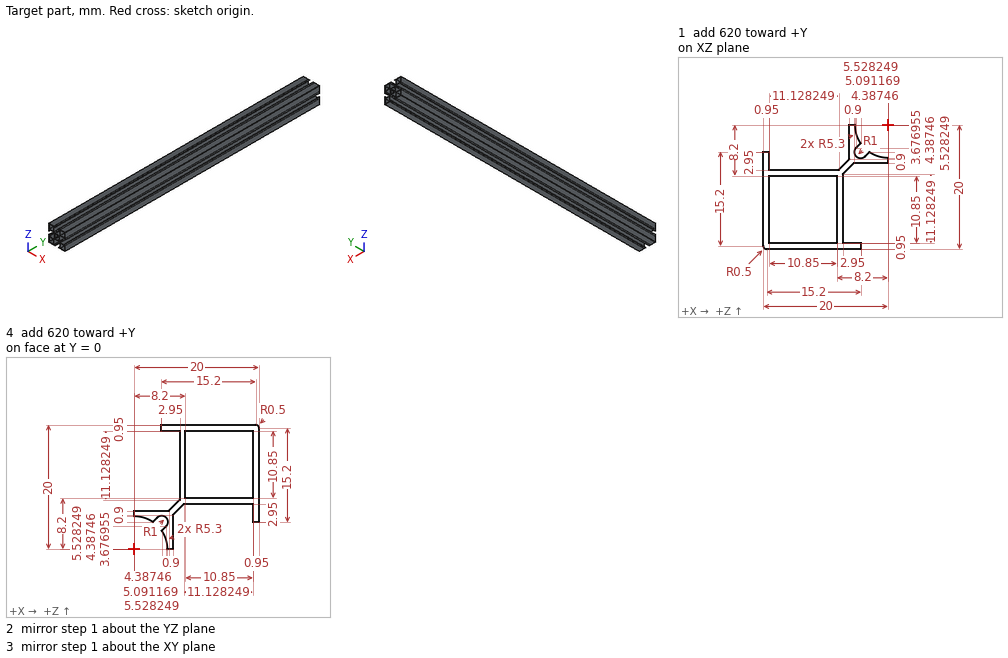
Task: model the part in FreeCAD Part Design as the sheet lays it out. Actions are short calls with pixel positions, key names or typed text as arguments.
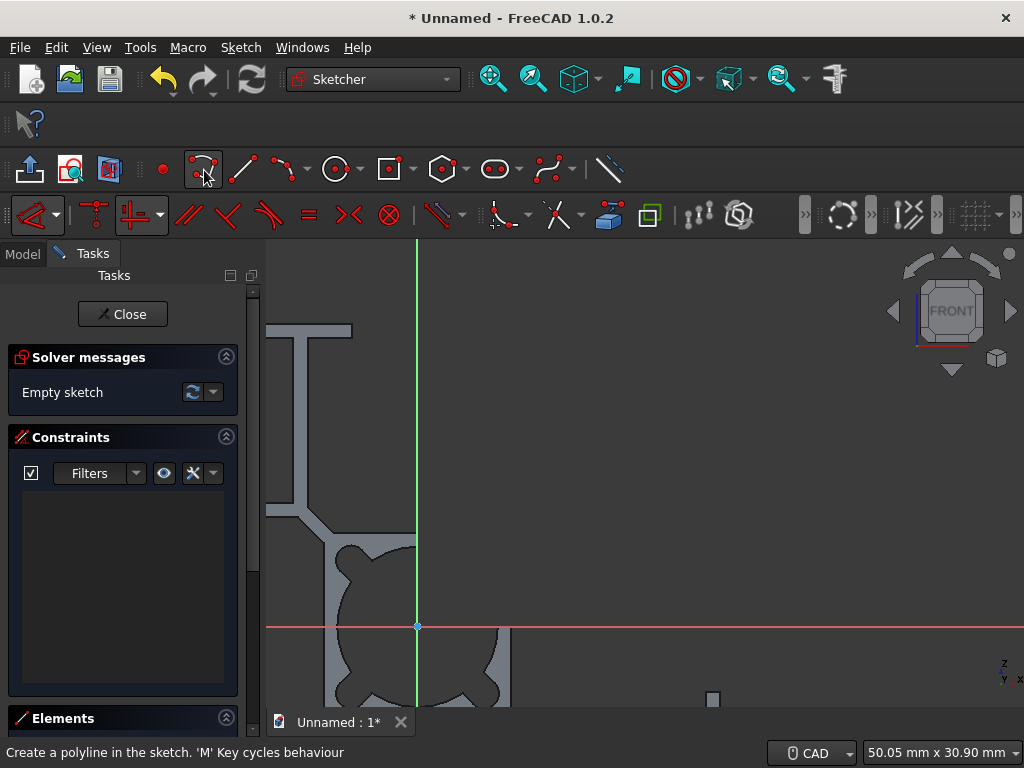
click(720, 332)
click(720, 562)
click(706, 562)
click(706, 517)
click(537, 517)
click(511, 543)
click(511, 627)
click(498, 618)
right_click(498, 618)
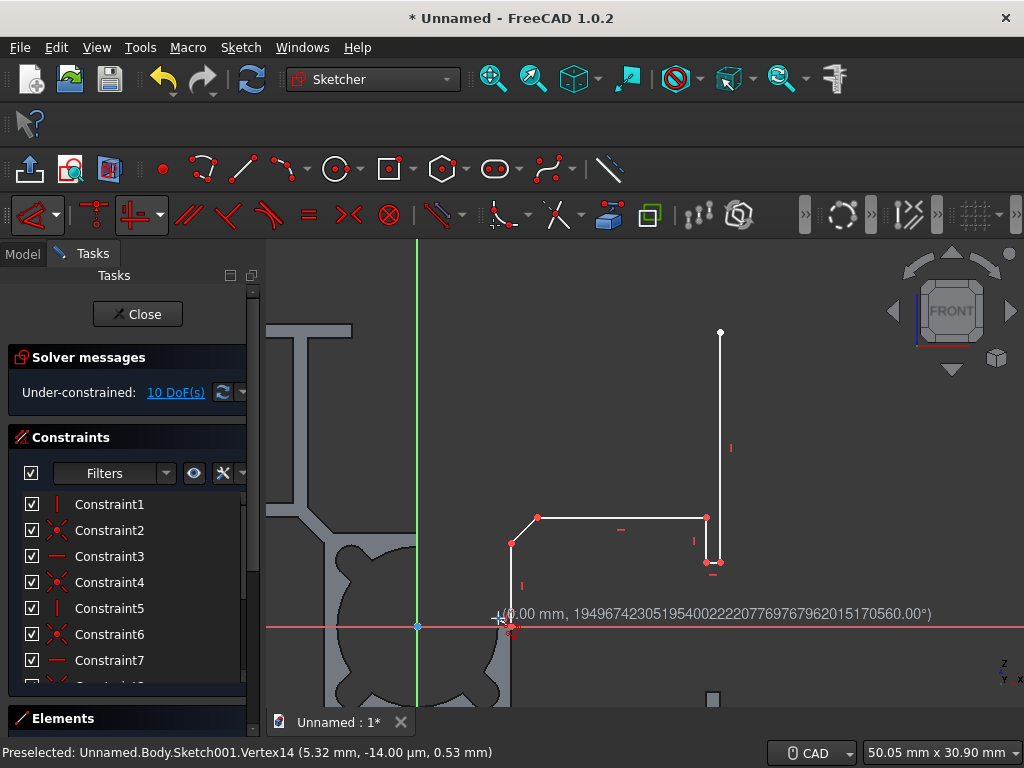
click(244, 170)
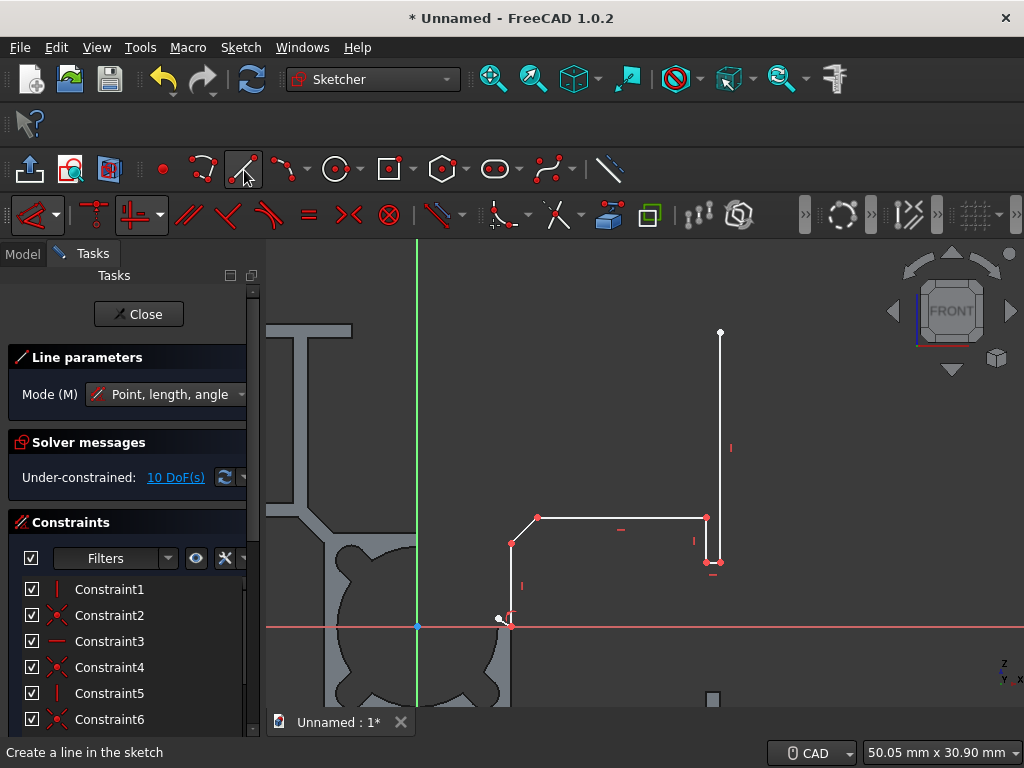
click(484, 582)
click(495, 571)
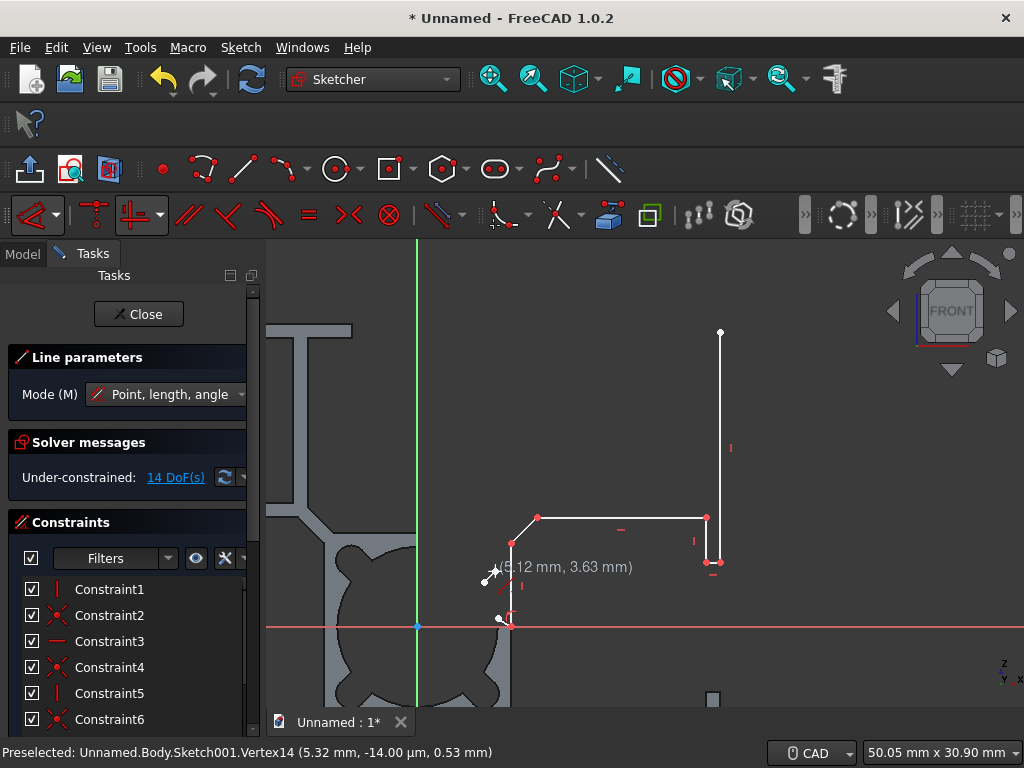
click(473, 550)
click(463, 561)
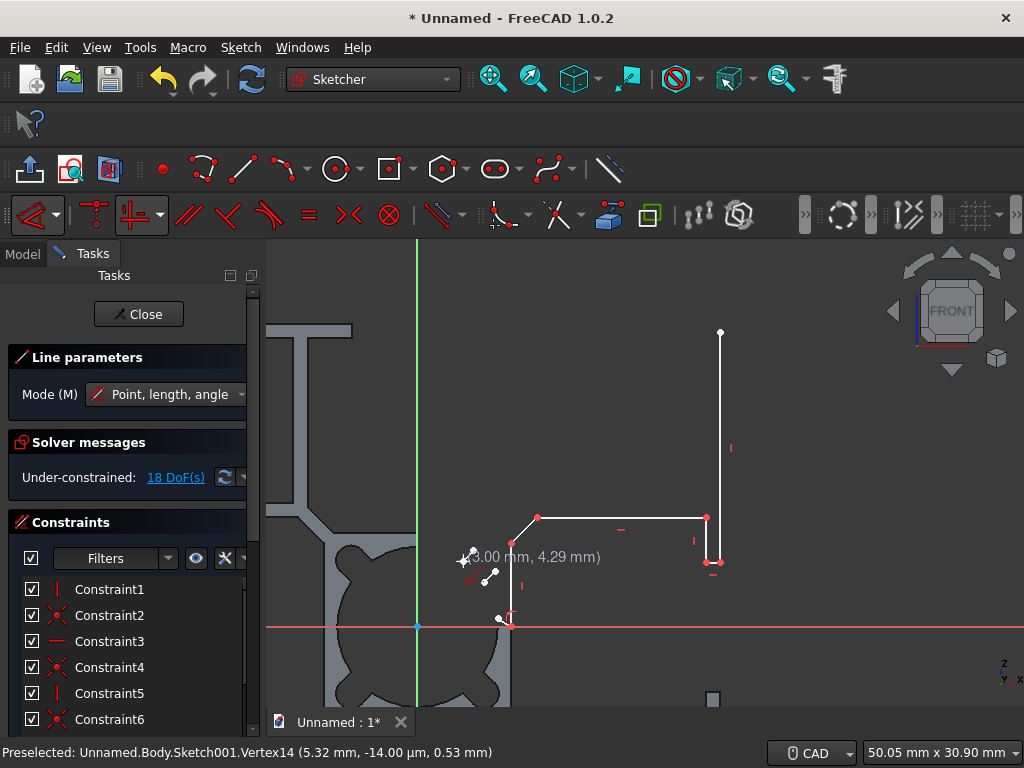
click(204, 170)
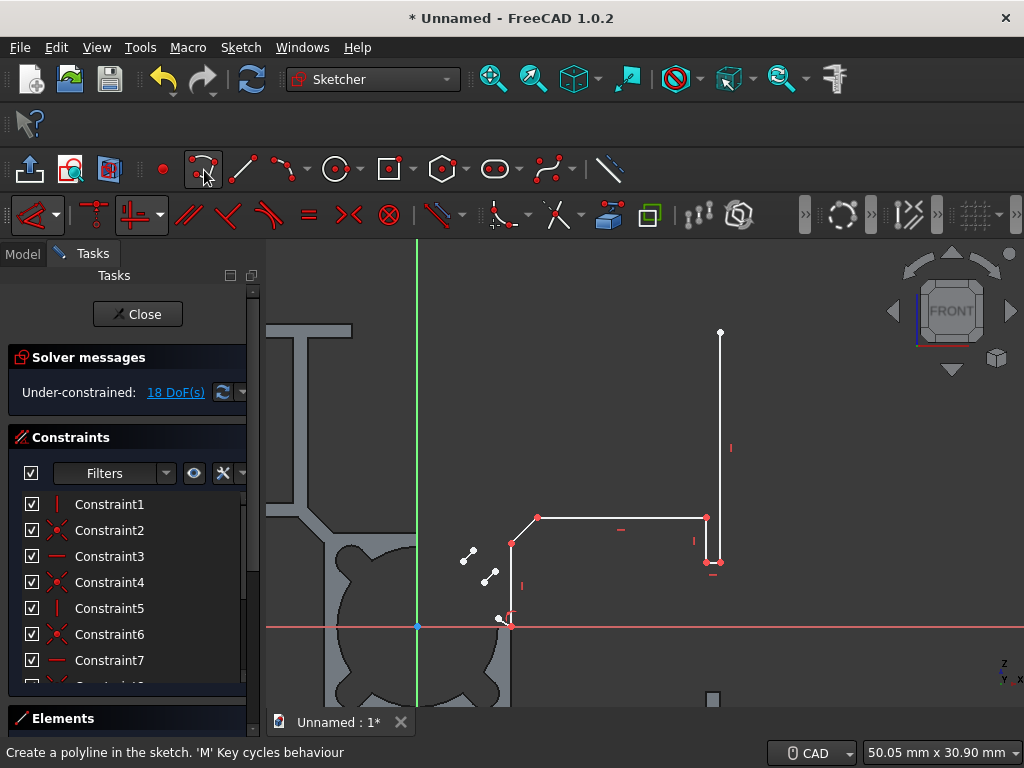
click(417, 547)
click(426, 533)
click(501, 533)
click(527, 507)
click(527, 338)
click(483, 338)
click(483, 324)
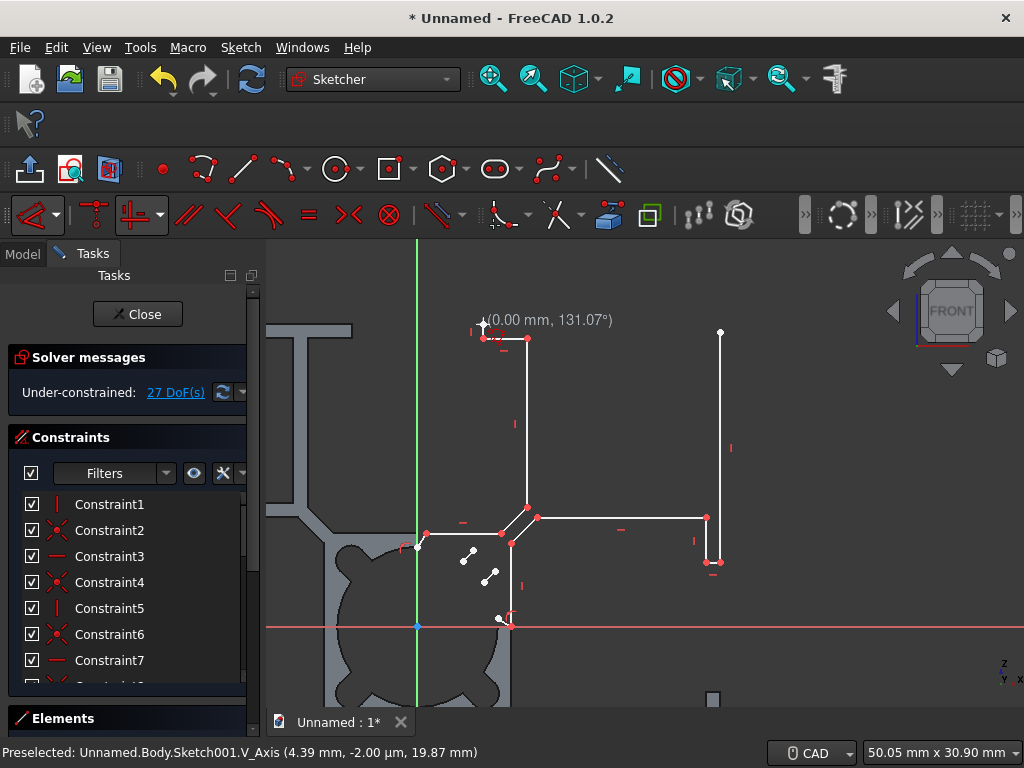
scroll(713, 324, up, 2)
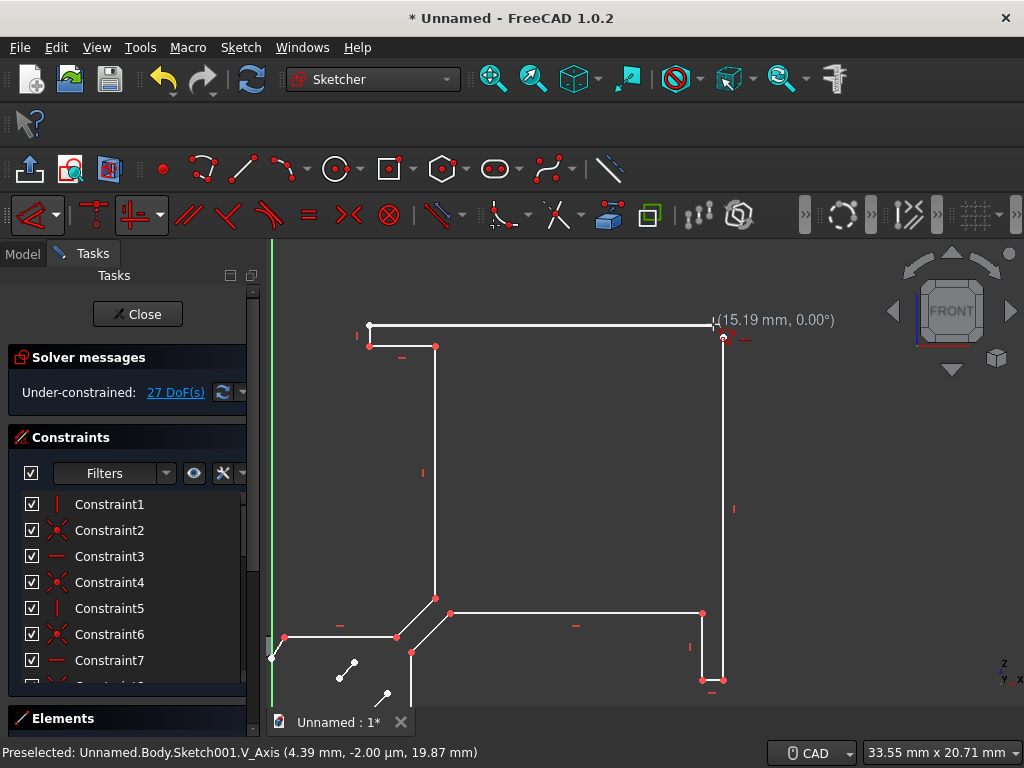
click(712, 324)
right_click(712, 324)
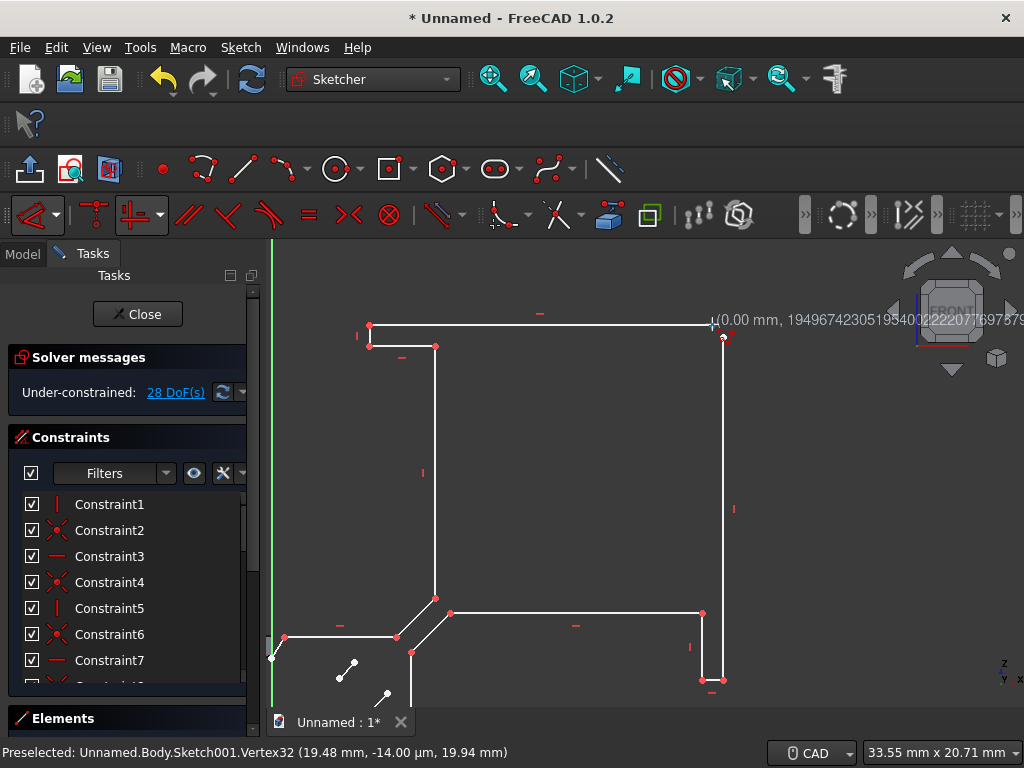
click(284, 170)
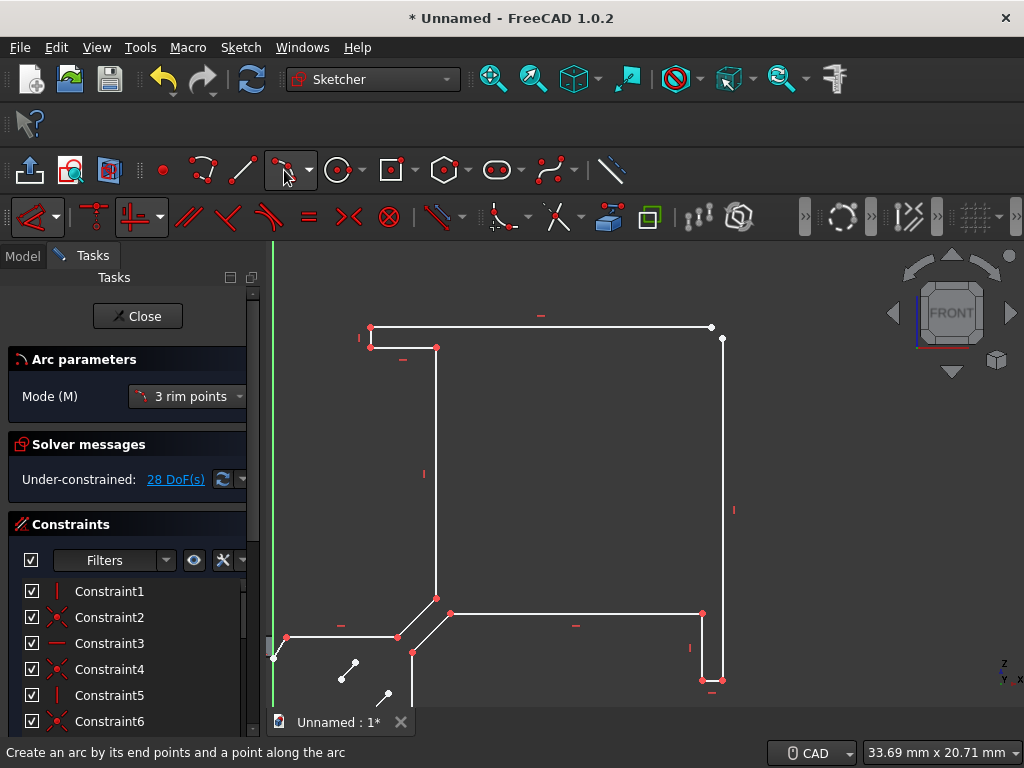
scroll(735, 318, down, 2)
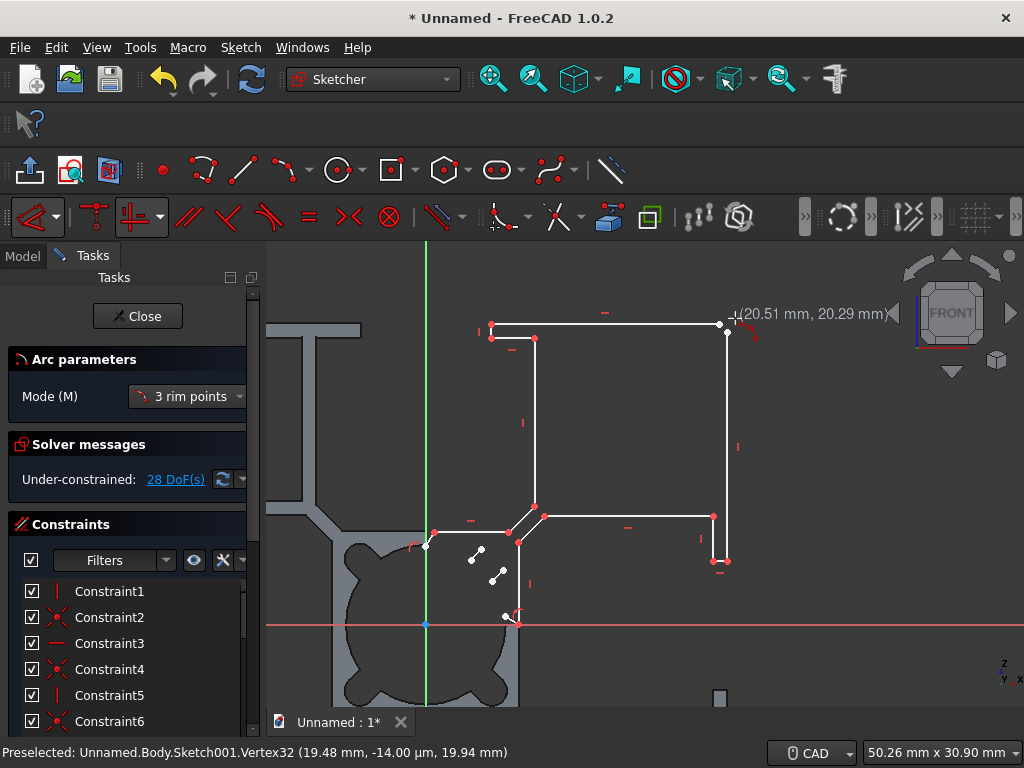
scroll(506, 625, up, 5)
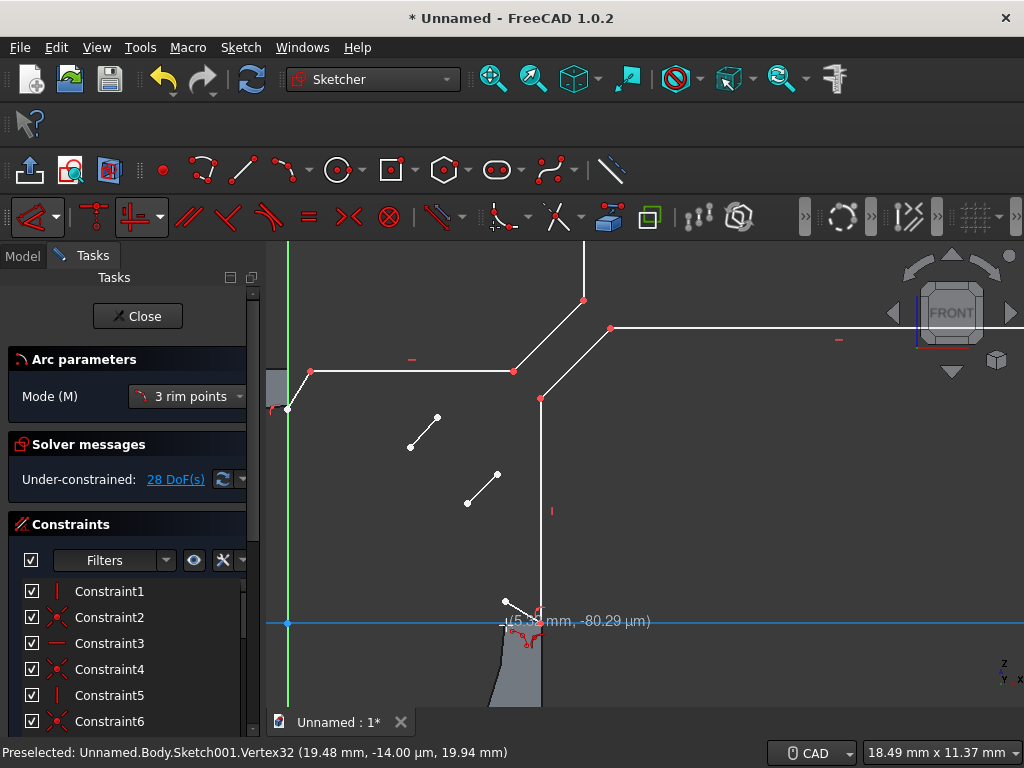
click(505, 601)
click(468, 504)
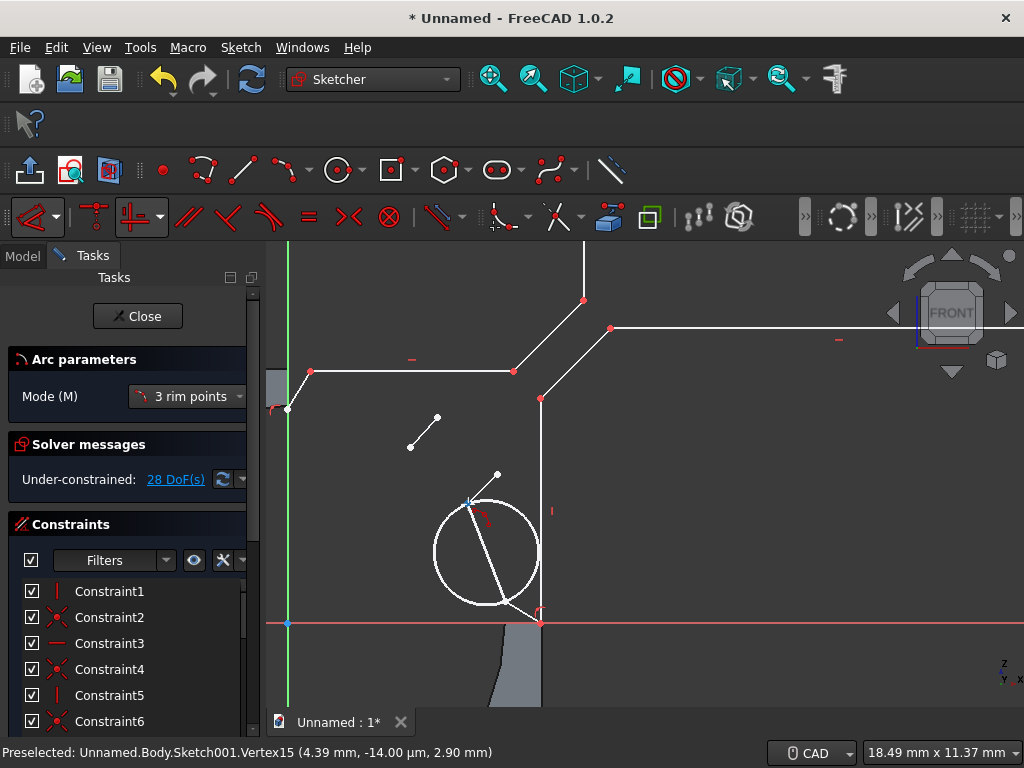
scroll(495, 559, up, 3)